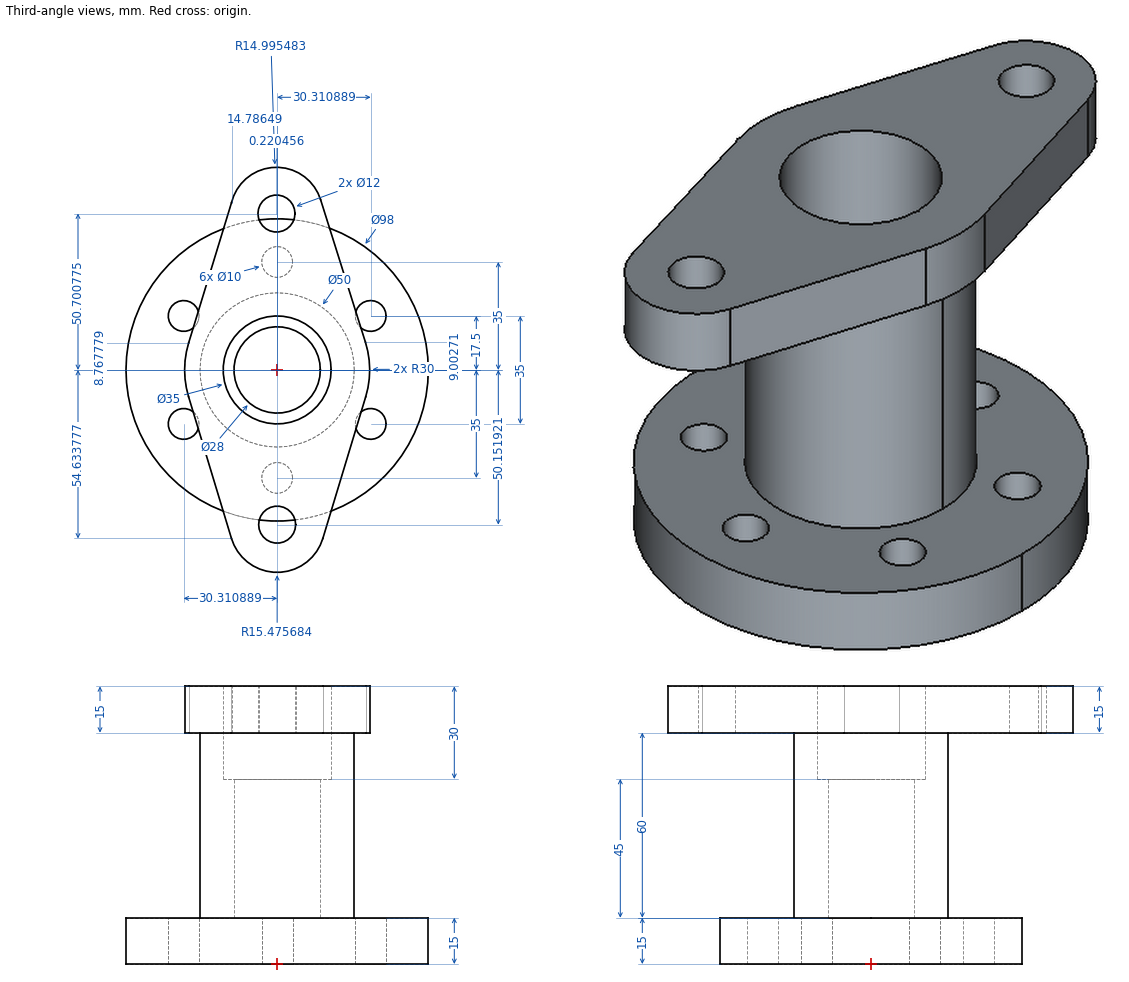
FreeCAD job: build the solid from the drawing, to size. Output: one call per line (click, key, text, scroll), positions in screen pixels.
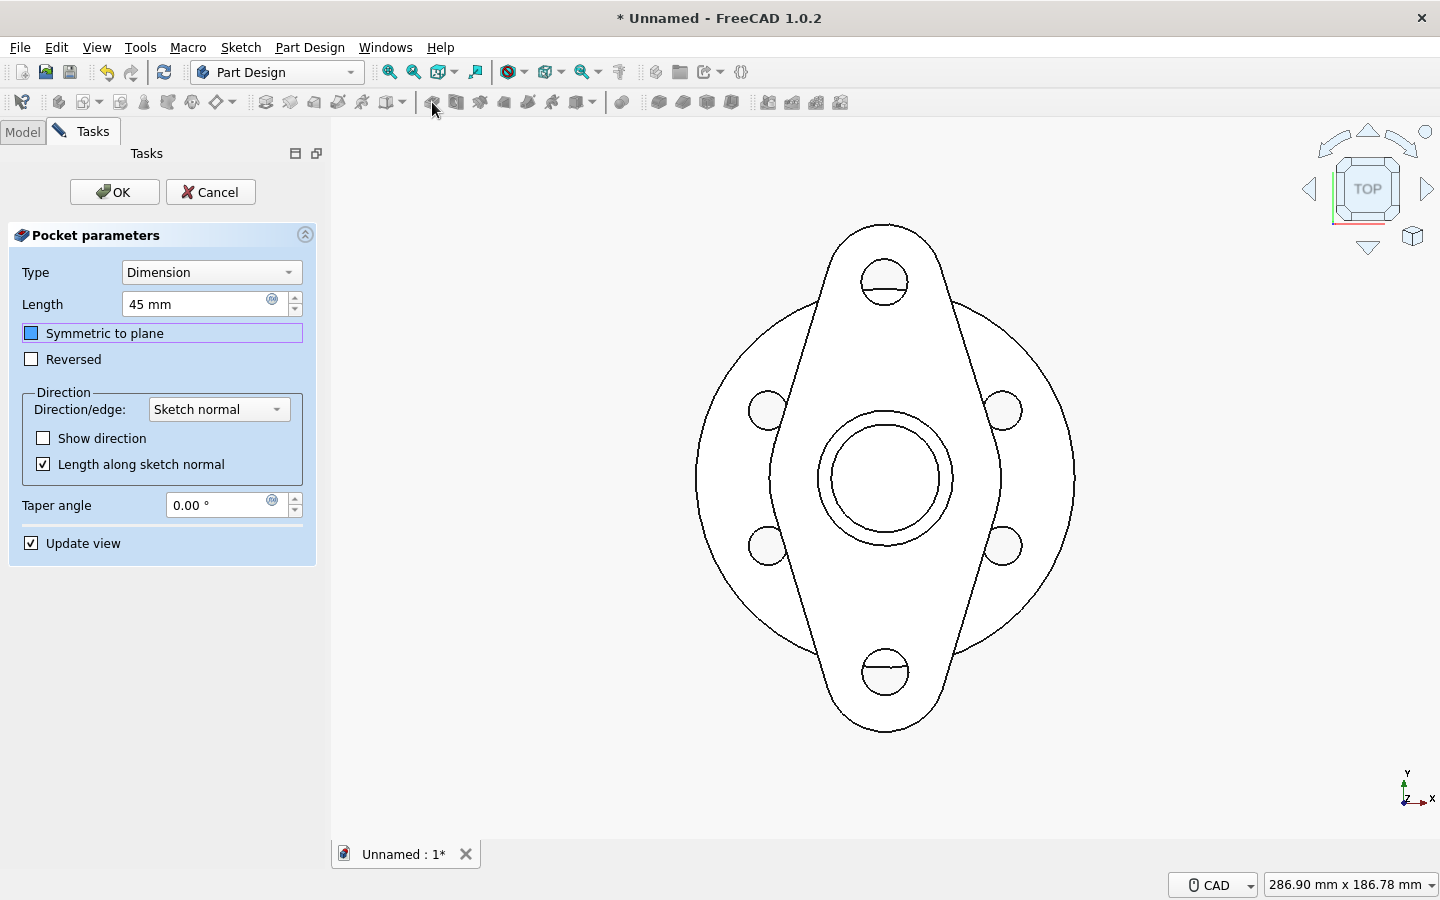
click(115, 192)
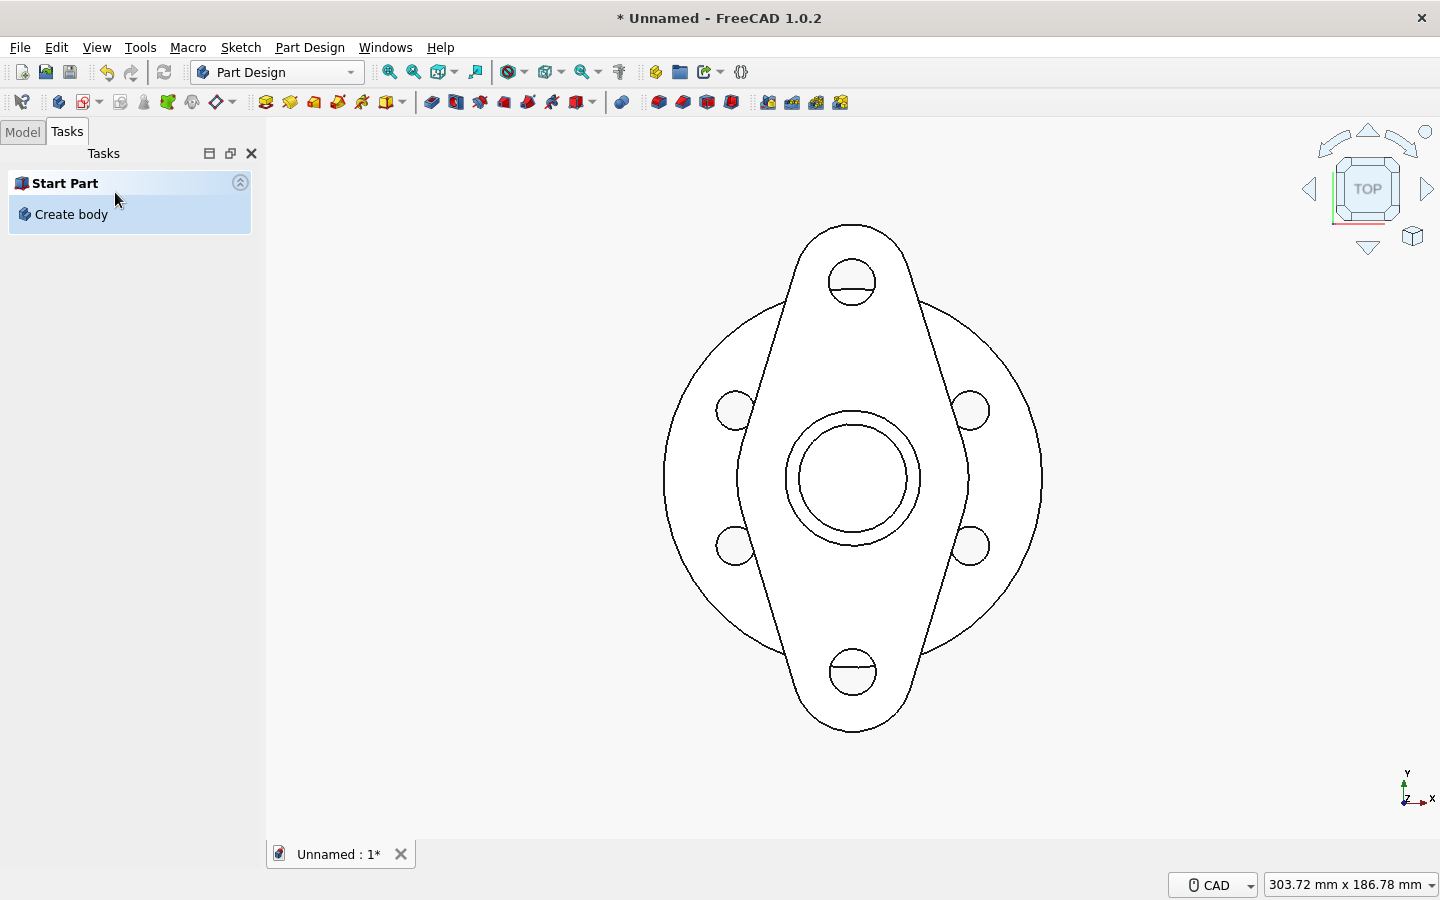
key(0)